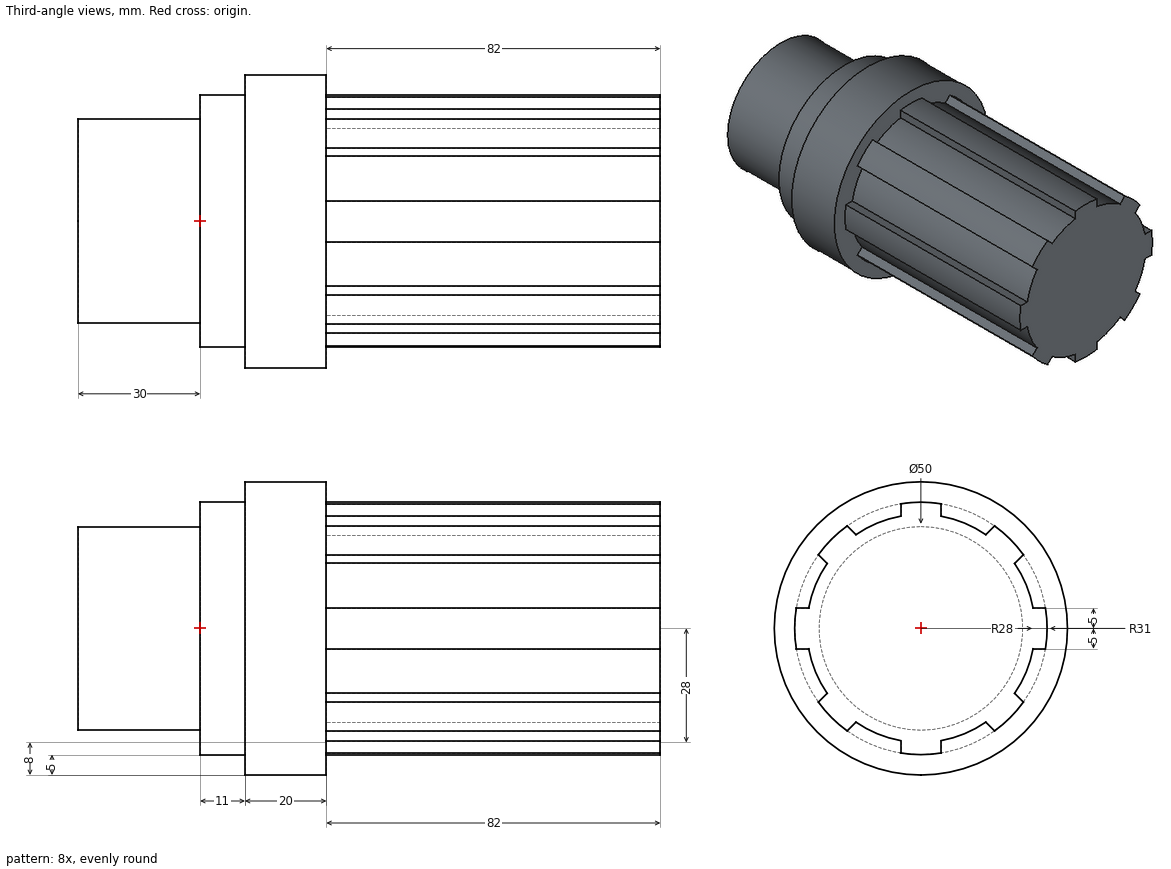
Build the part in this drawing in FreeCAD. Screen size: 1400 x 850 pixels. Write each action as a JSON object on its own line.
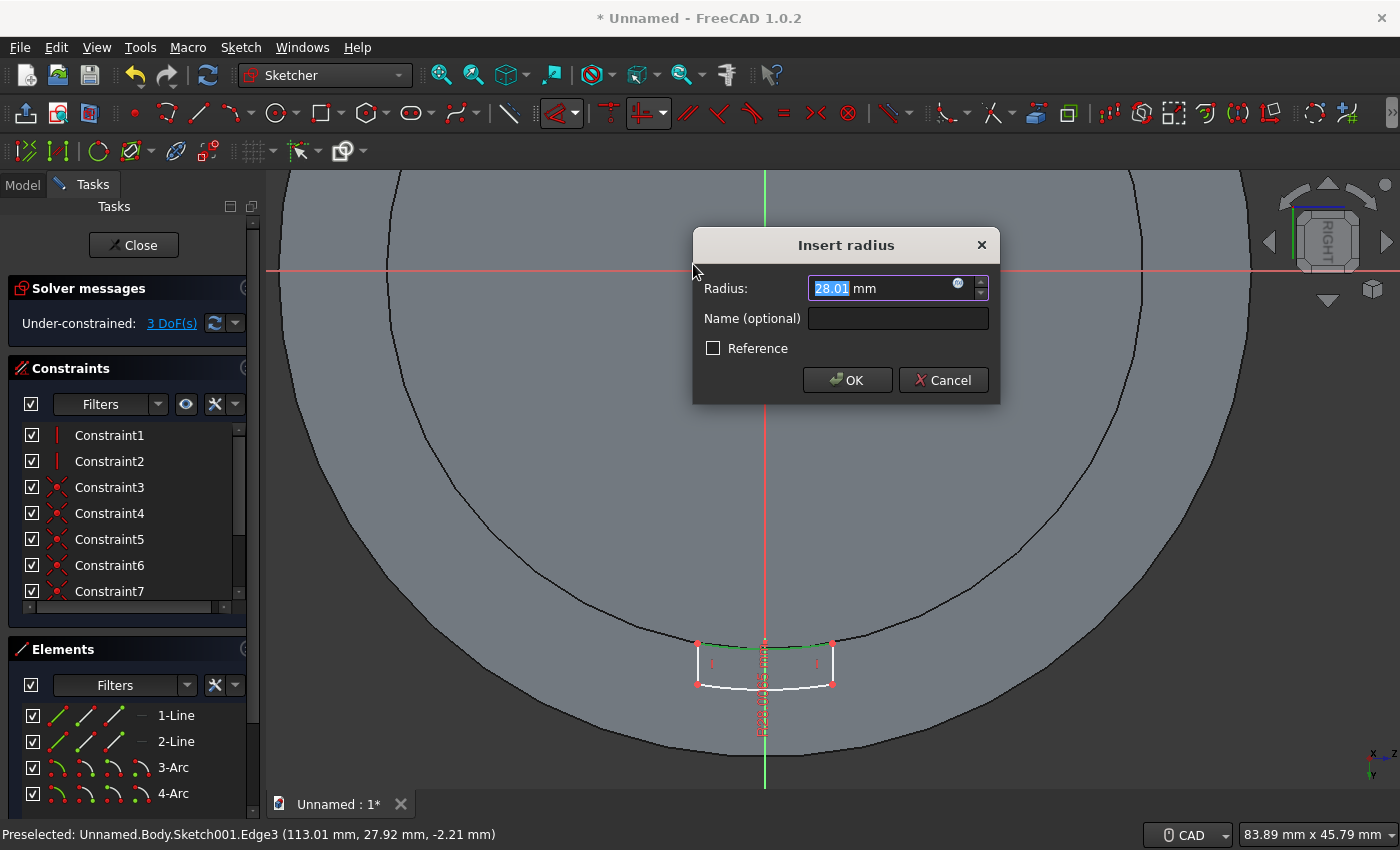
{"action": "type", "text": "28"}
{"action": "key", "text": "Return"}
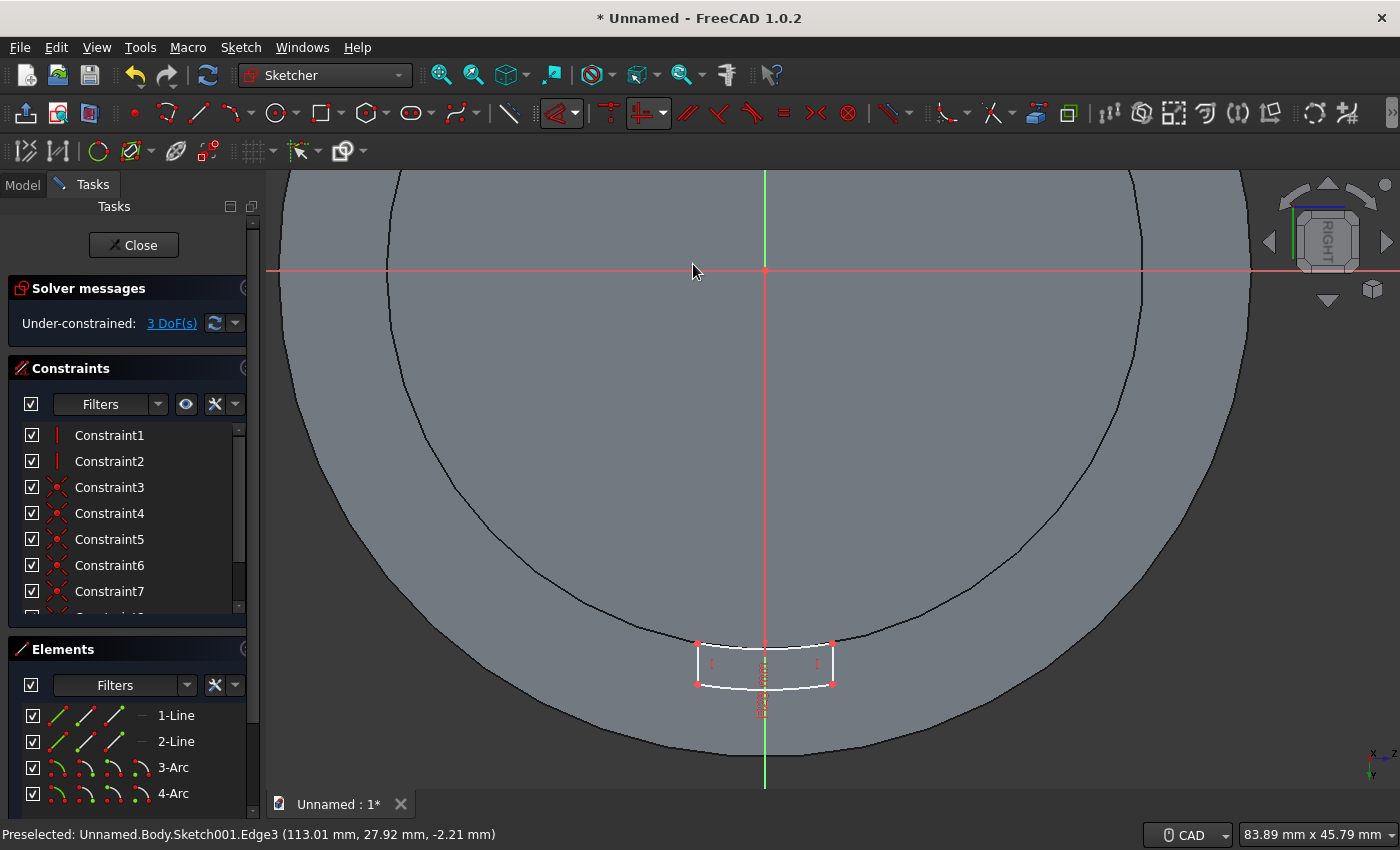
{"action": "left_click", "coordinate": [738, 689]}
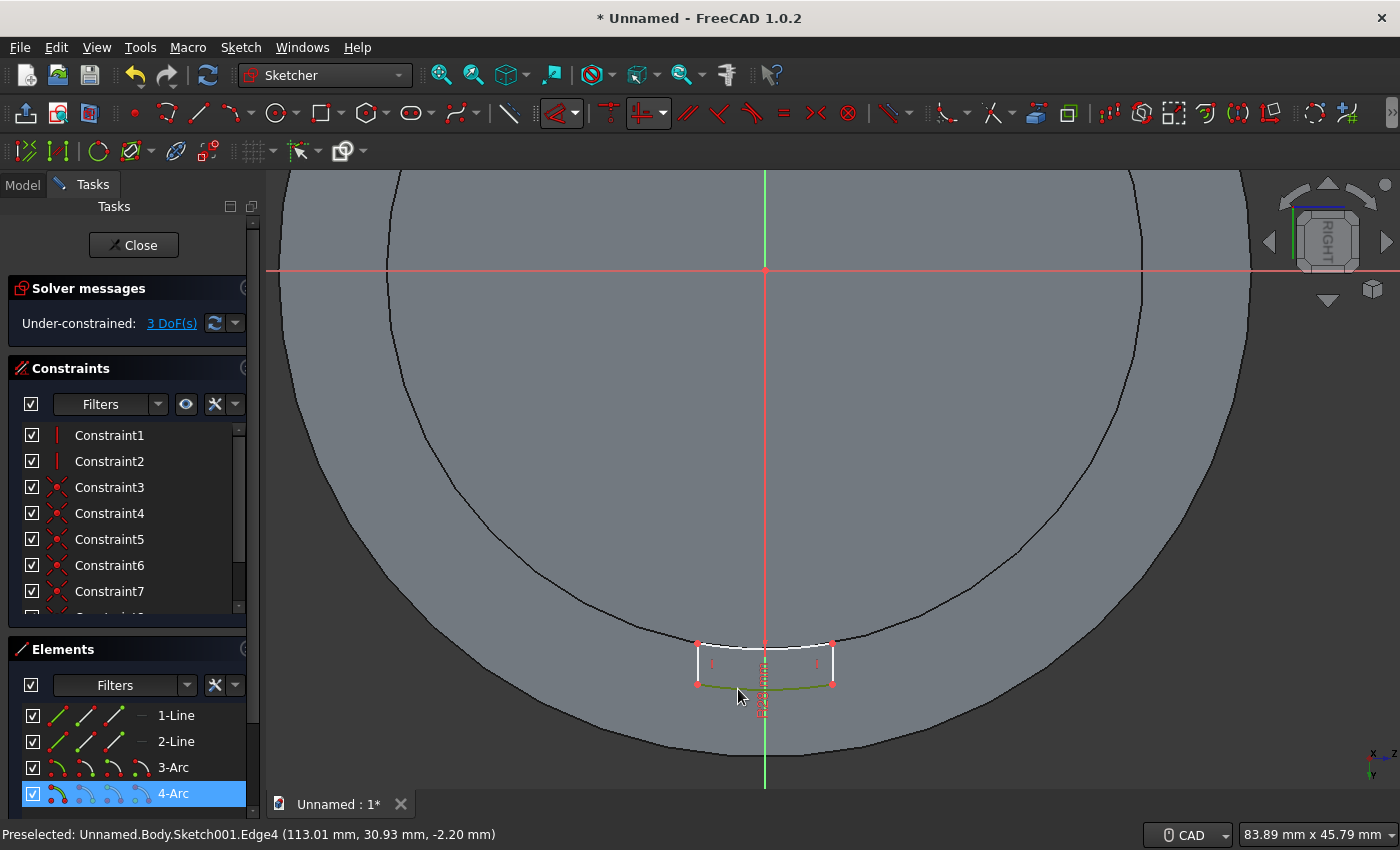
{"action": "left_click", "coordinate": [578, 114]}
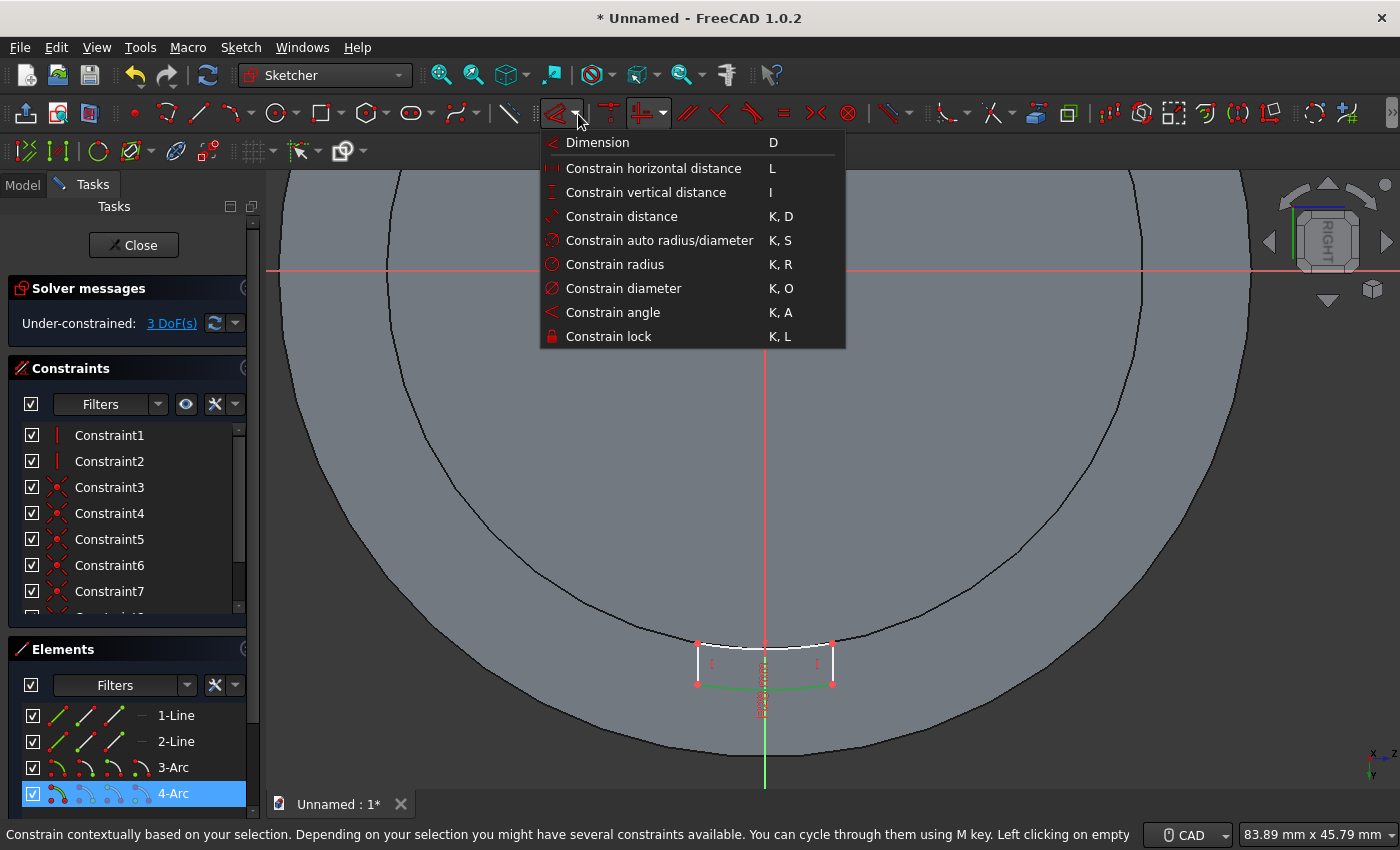
{"action": "left_click", "coordinate": [693, 264]}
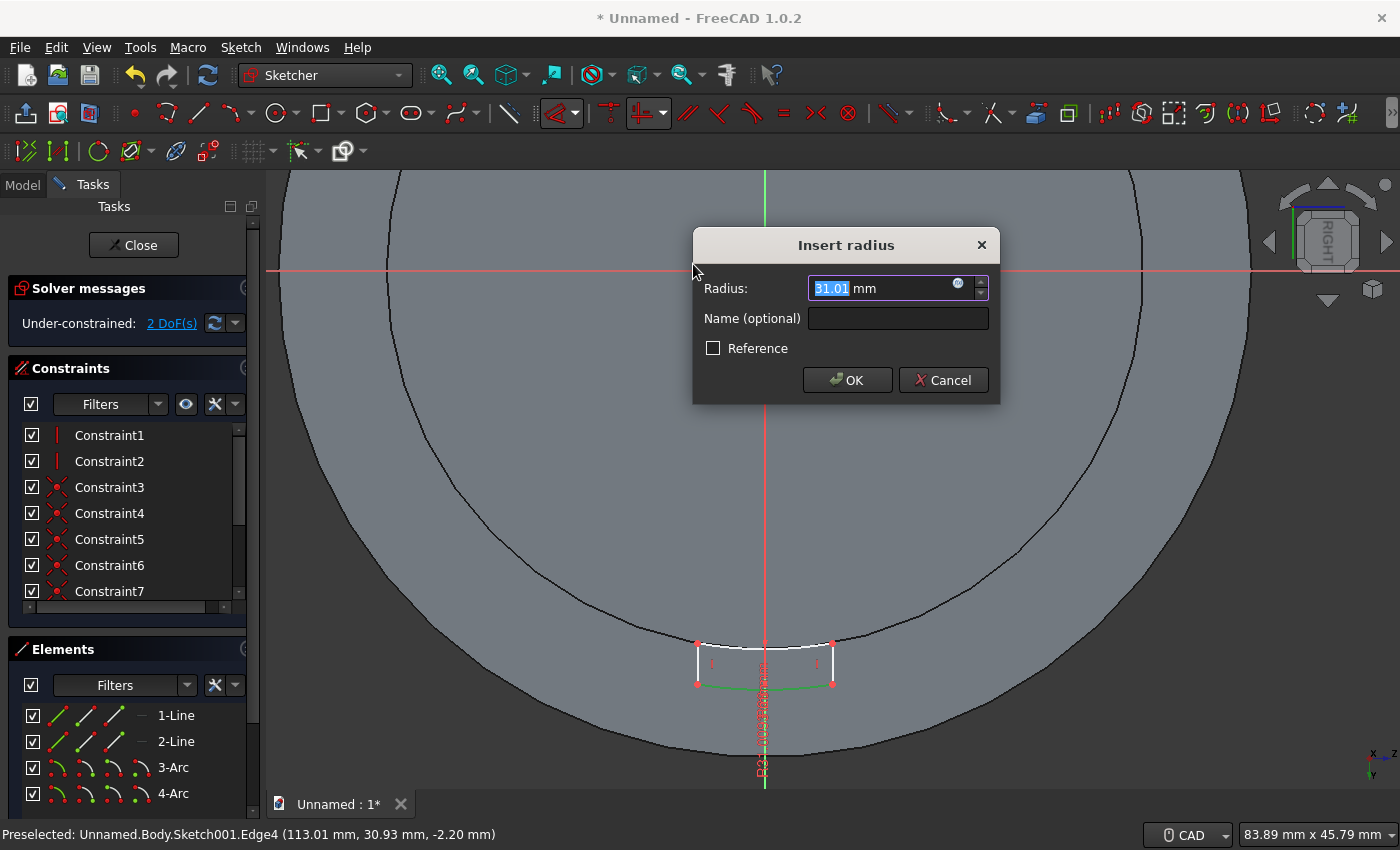
{"action": "type", "text": "31"}
{"action": "key", "text": "Return"}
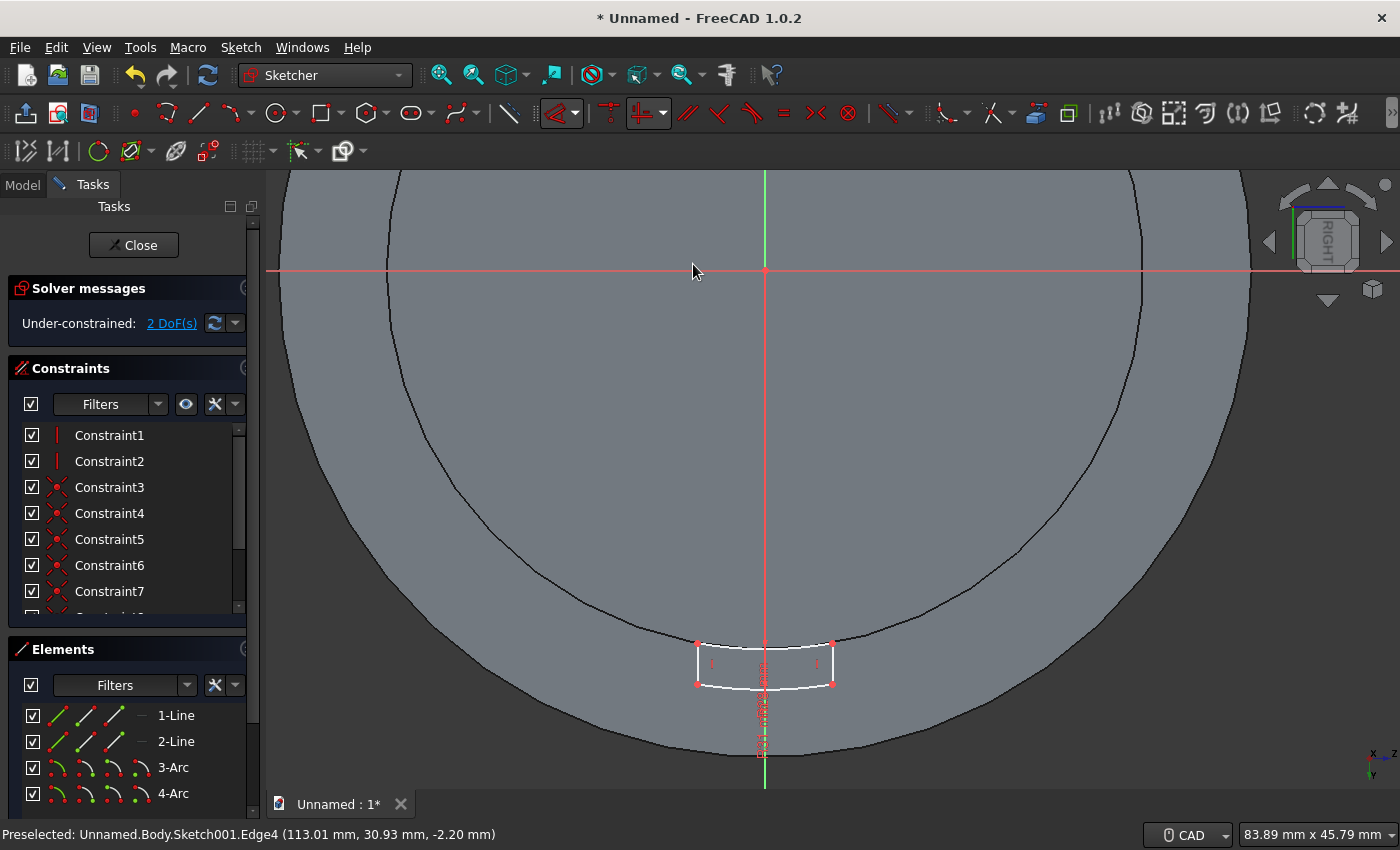
{"action": "left_click", "coordinate": [833, 684]}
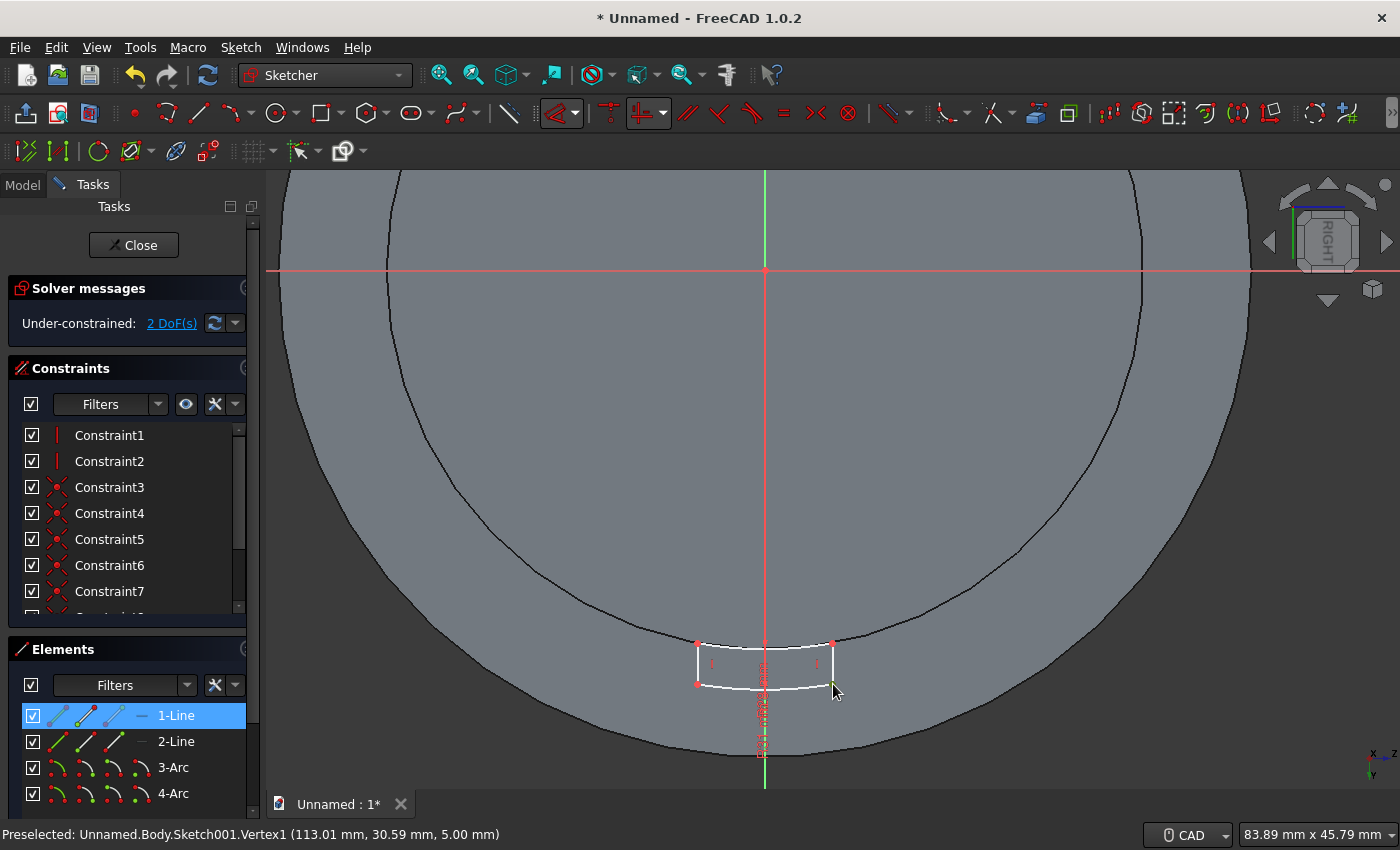
{"action": "key", "text": "l"}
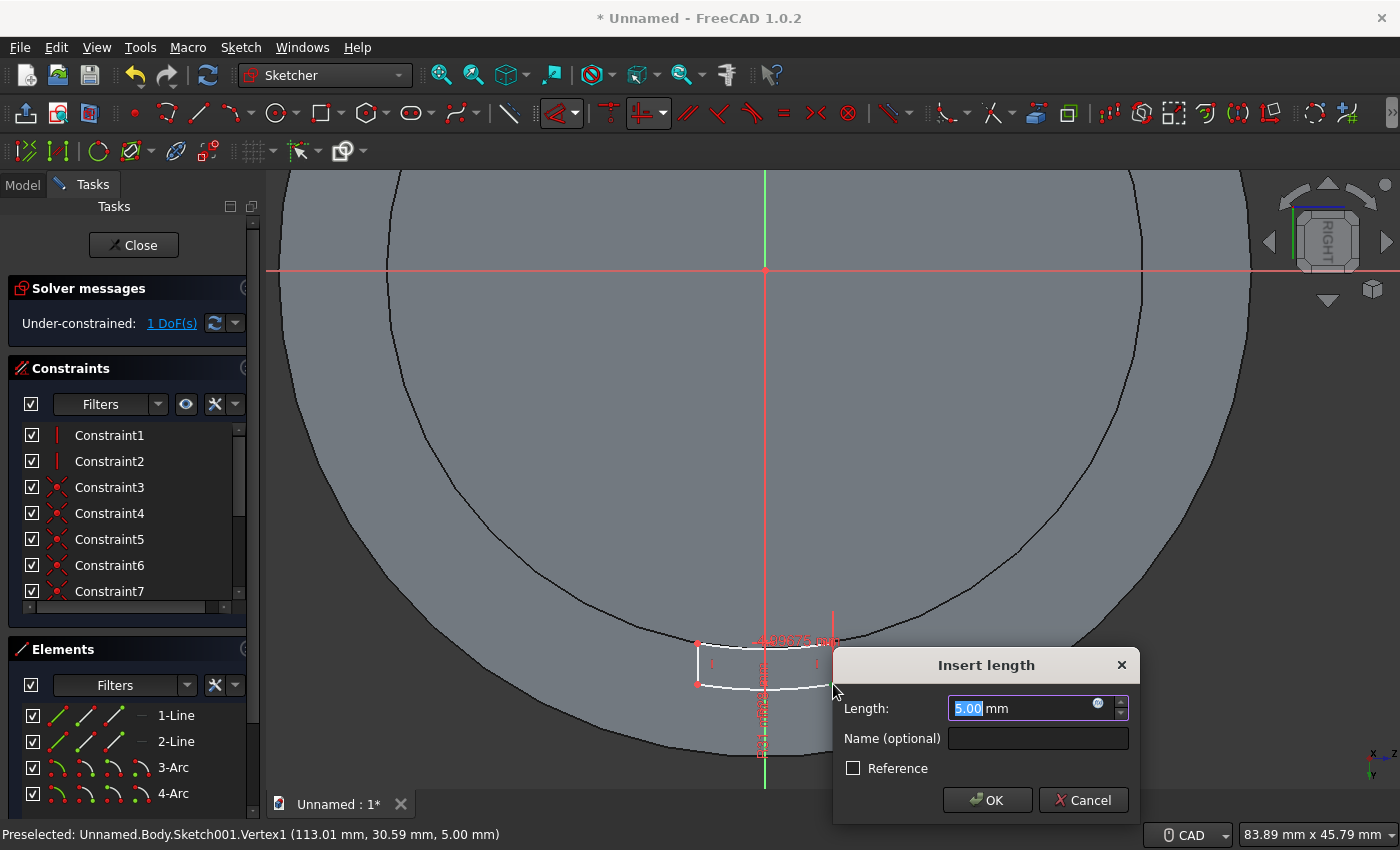
{"action": "type", "text": "5"}
{"action": "key", "text": "Return"}